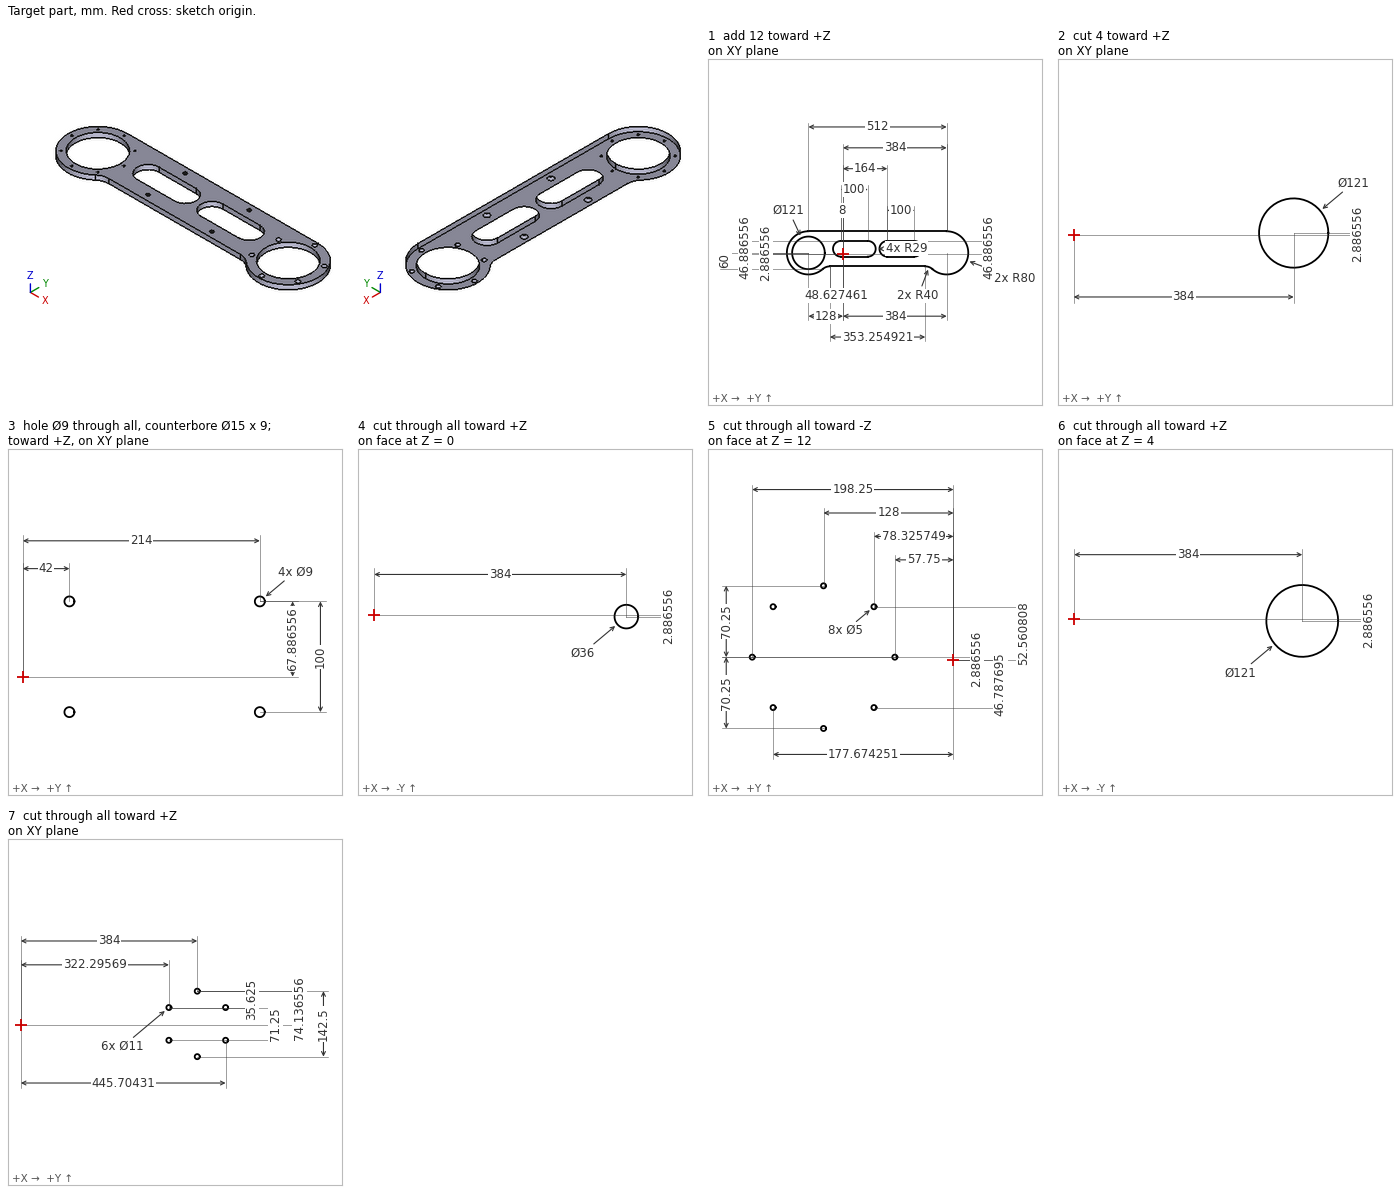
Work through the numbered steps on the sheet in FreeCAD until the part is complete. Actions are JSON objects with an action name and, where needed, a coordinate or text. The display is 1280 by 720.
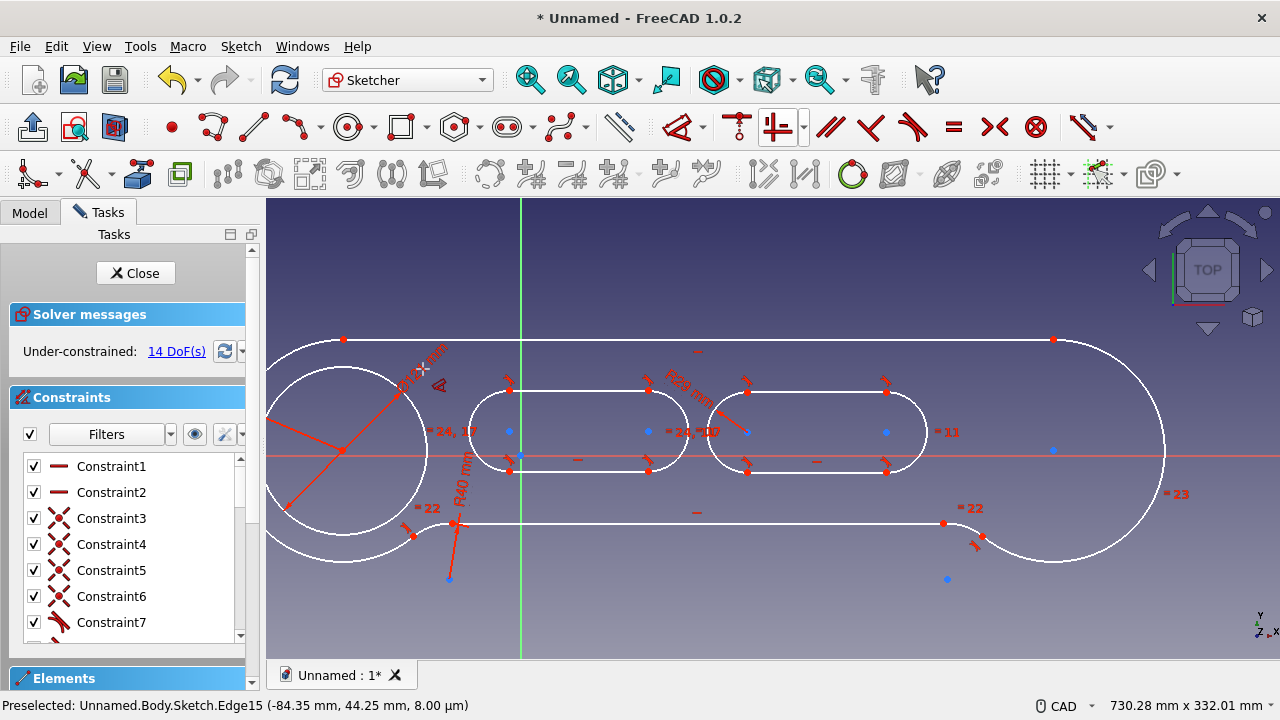
{"action": "scroll", "coordinate": [509, 391], "scroll_direction": "up", "scroll_amount": 7}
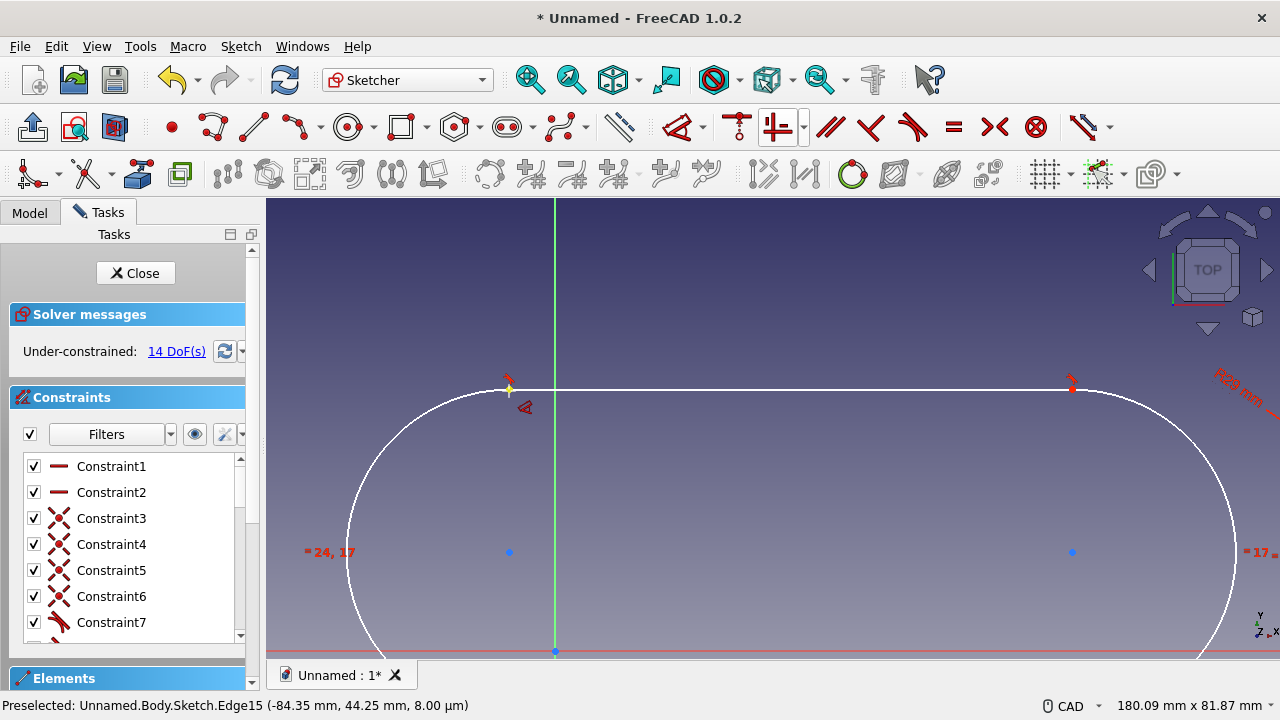
{"action": "left_click", "coordinate": [510, 390]}
{"action": "left_click", "coordinate": [533, 356]}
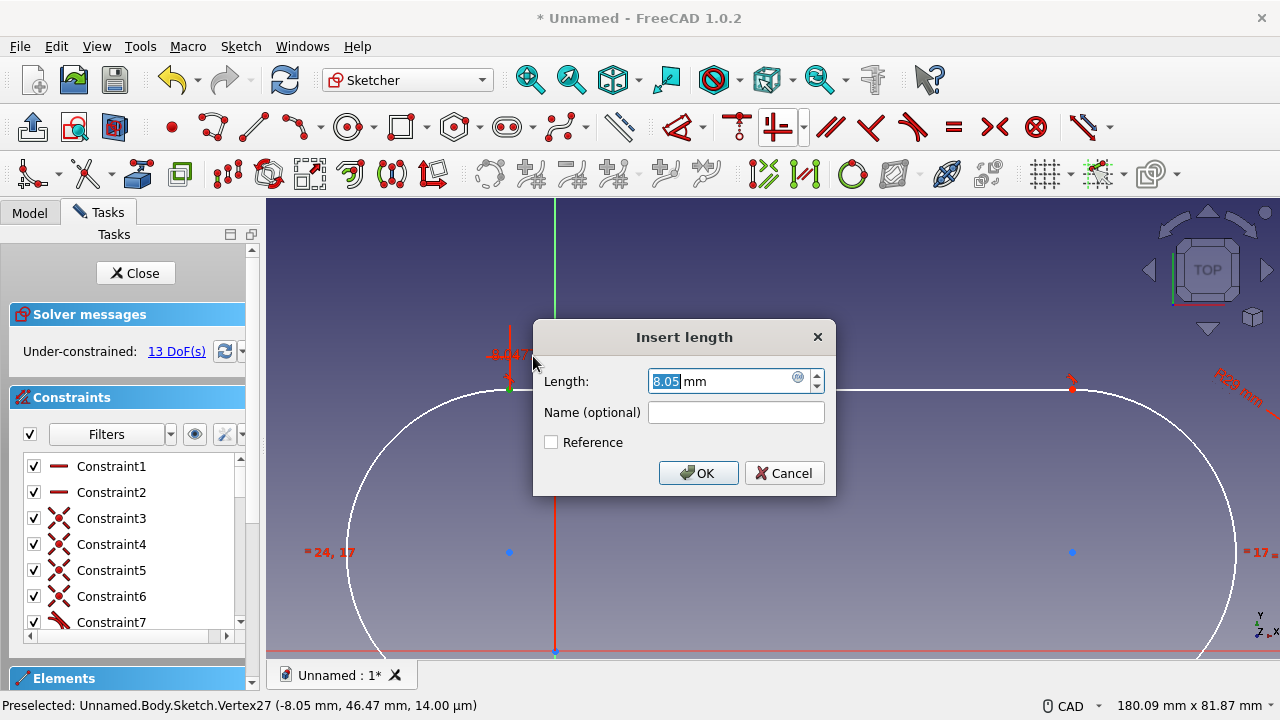
{"action": "type", "text": "8"}
{"action": "key", "text": "Return"}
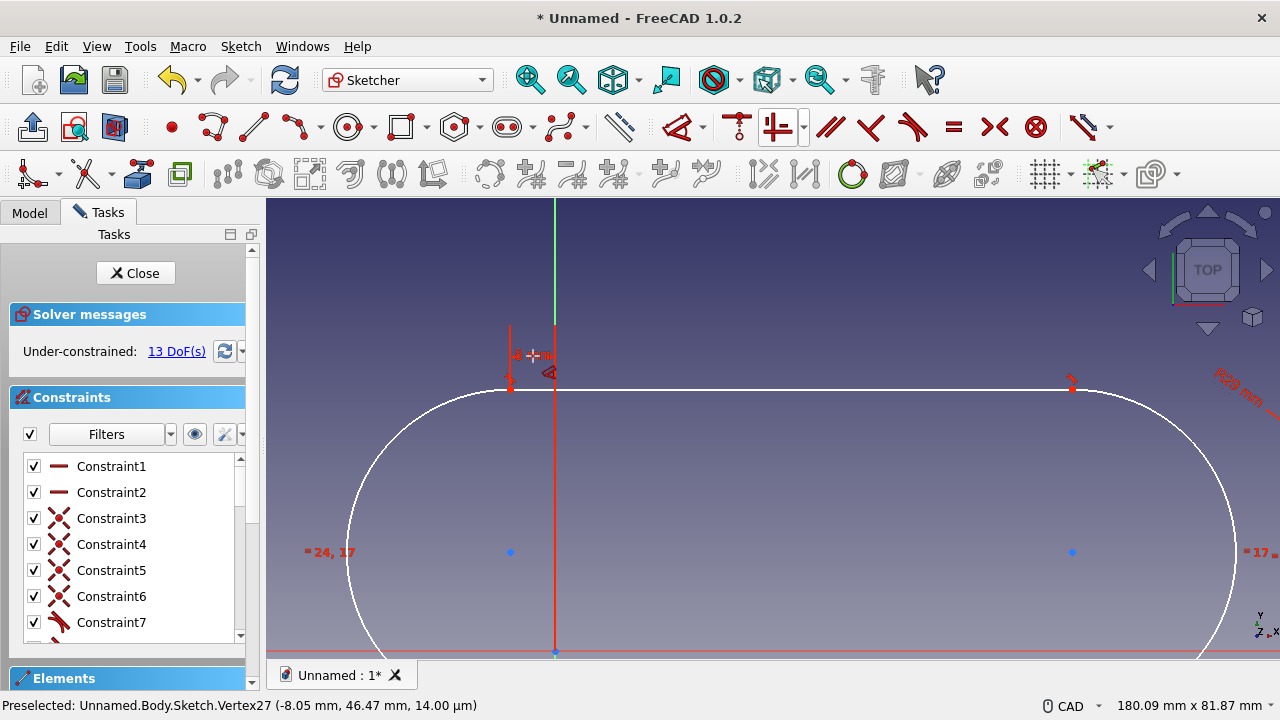
{"action": "scroll", "coordinate": [591, 398], "scroll_direction": "down", "scroll_amount": 9}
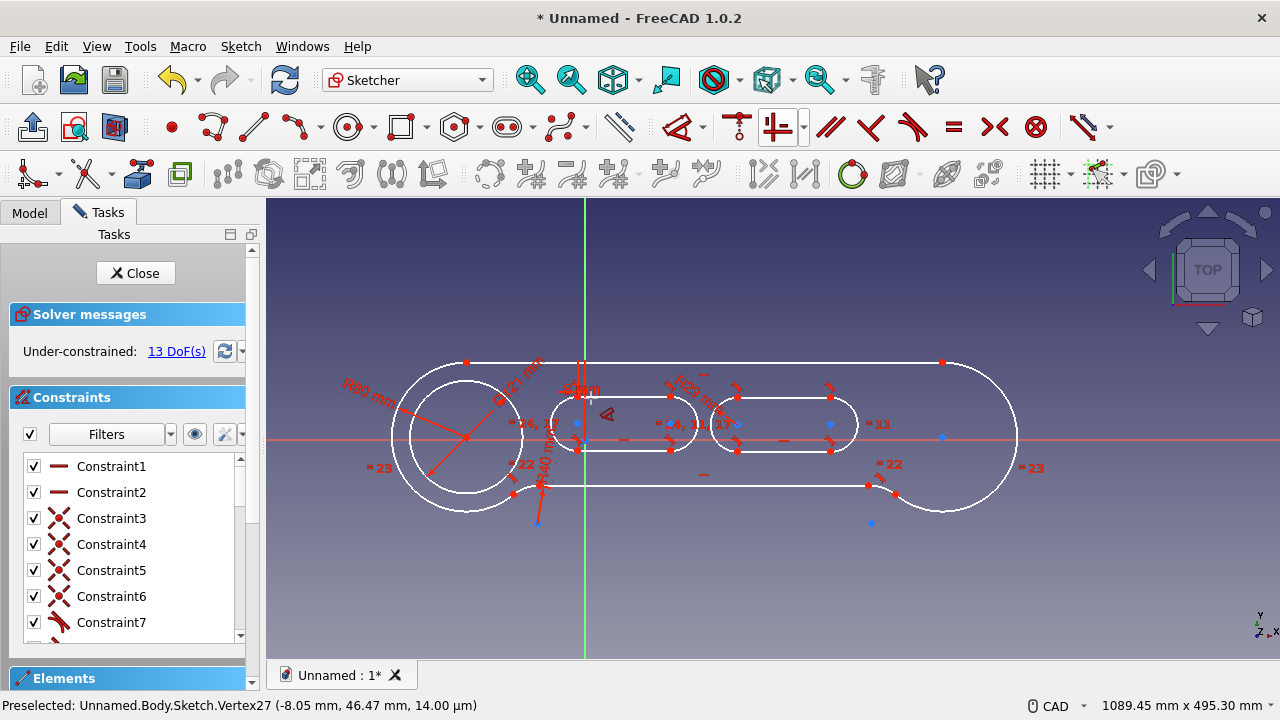
{"action": "left_click", "coordinate": [800, 363]}
{"action": "left_click", "coordinate": [705, 329]}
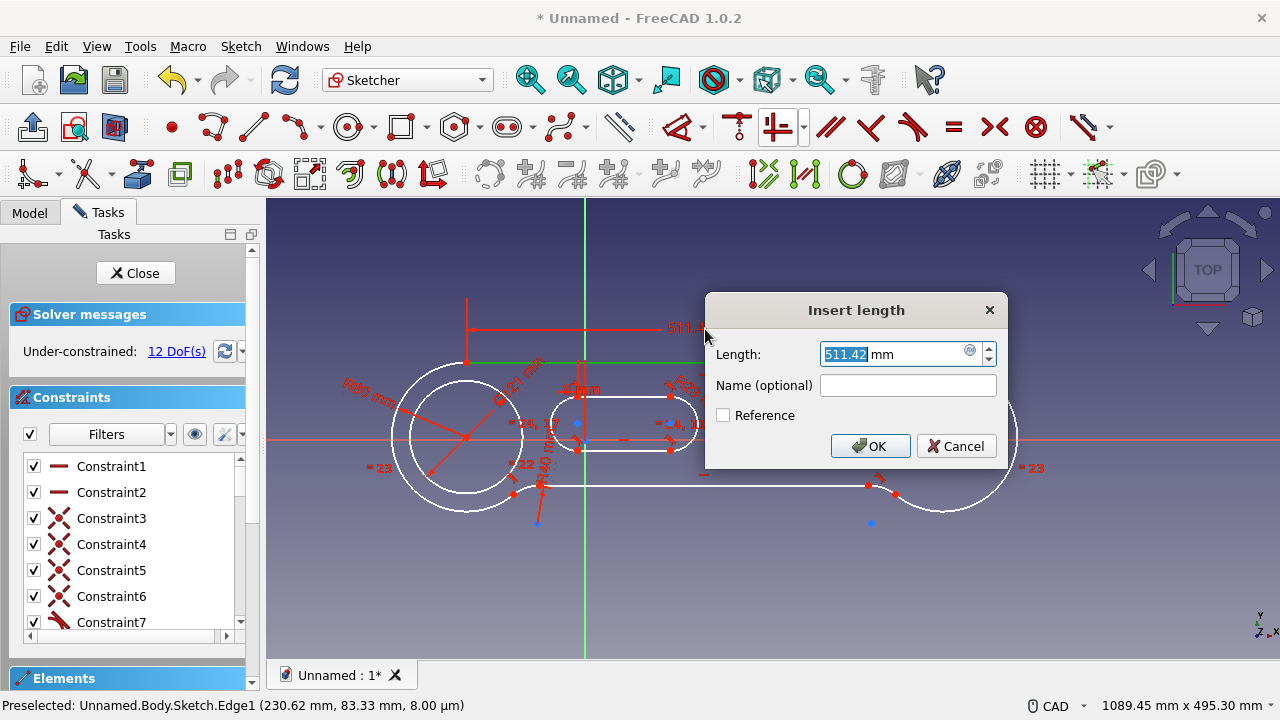
{"action": "type", "text": "512"}
{"action": "key", "text": "Return"}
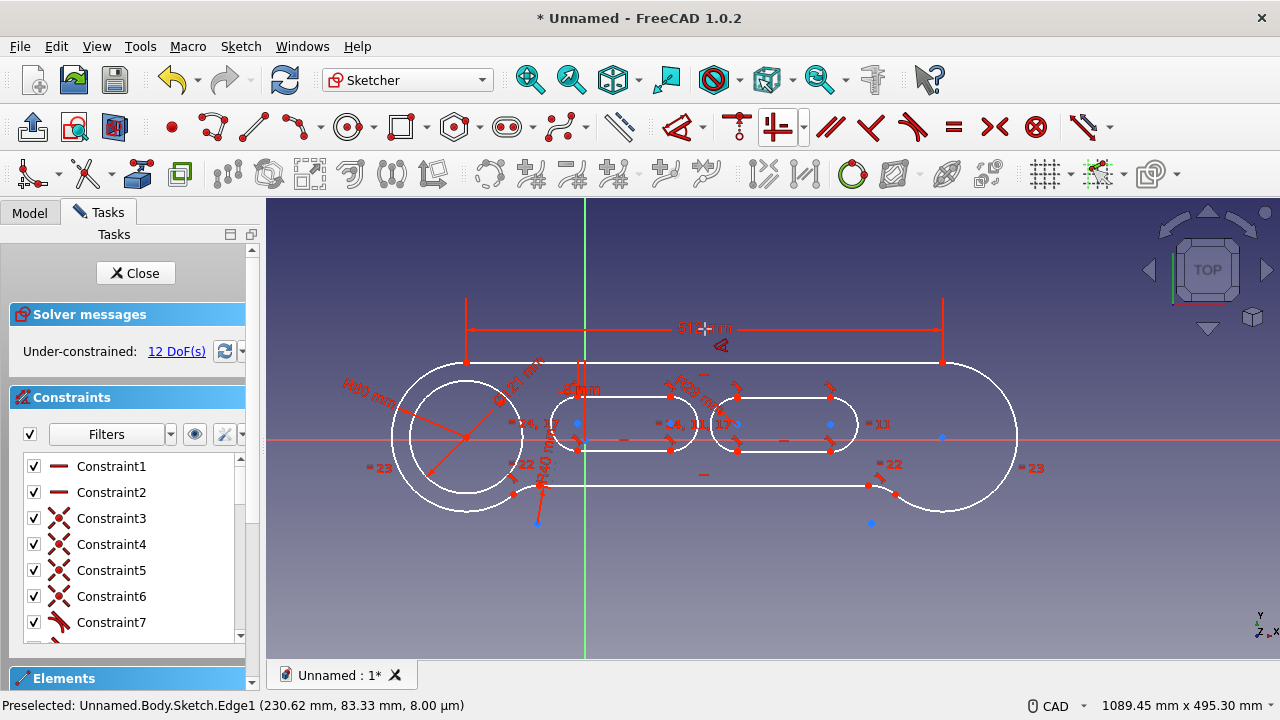
{"action": "left_click", "coordinate": [766, 398]}
{"action": "left_click", "coordinate": [784, 340]}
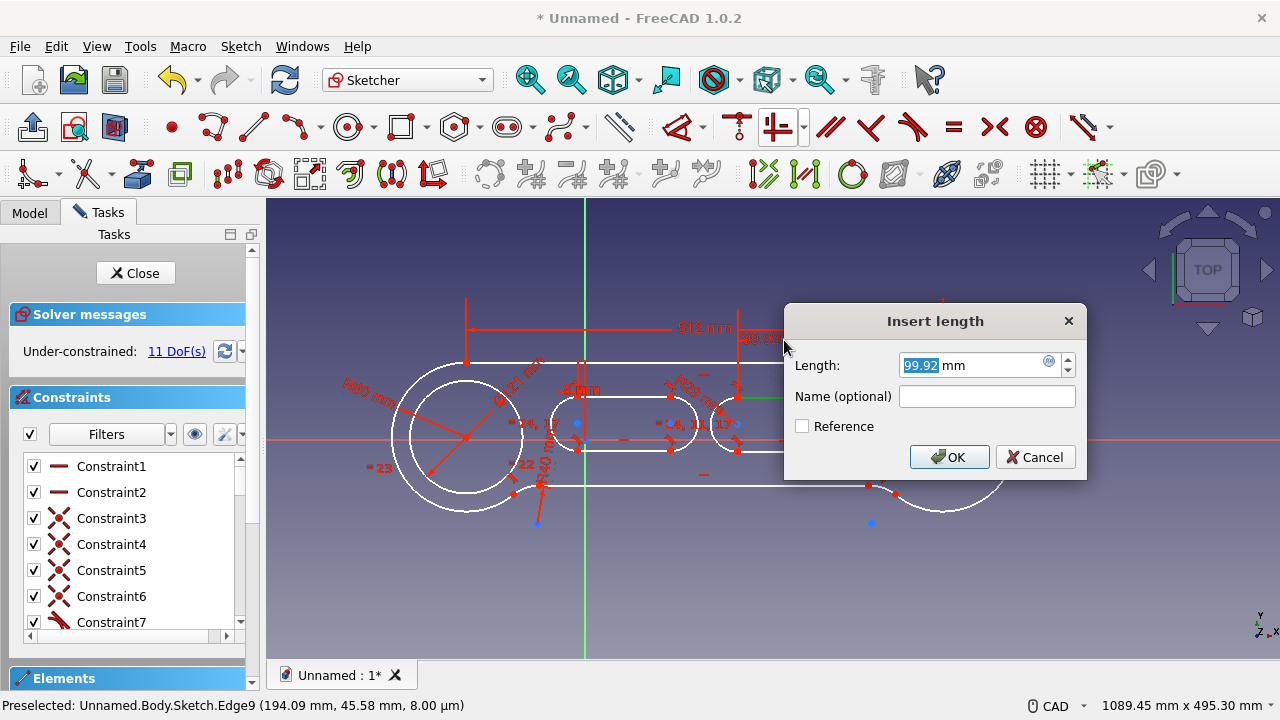
{"action": "type", "text": "100"}
{"action": "key", "text": "Return"}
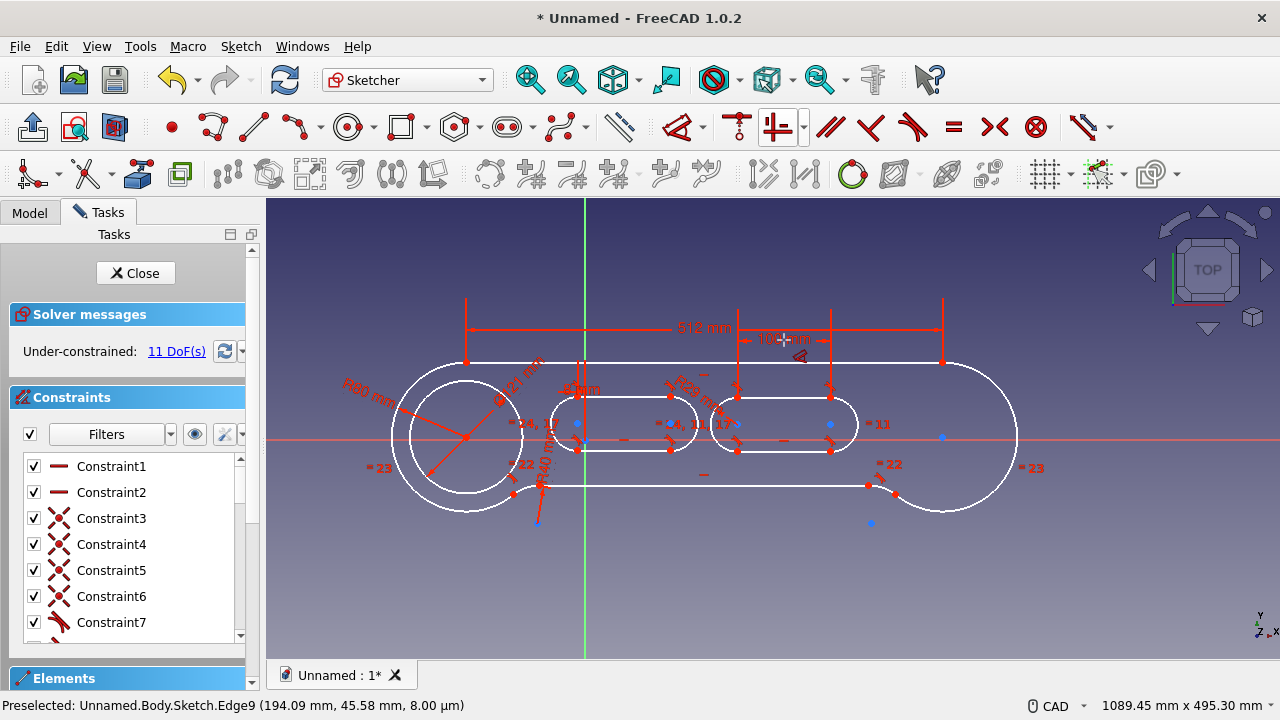
{"action": "left_click", "coordinate": [606, 397]}
{"action": "left_click", "coordinate": [624, 339]}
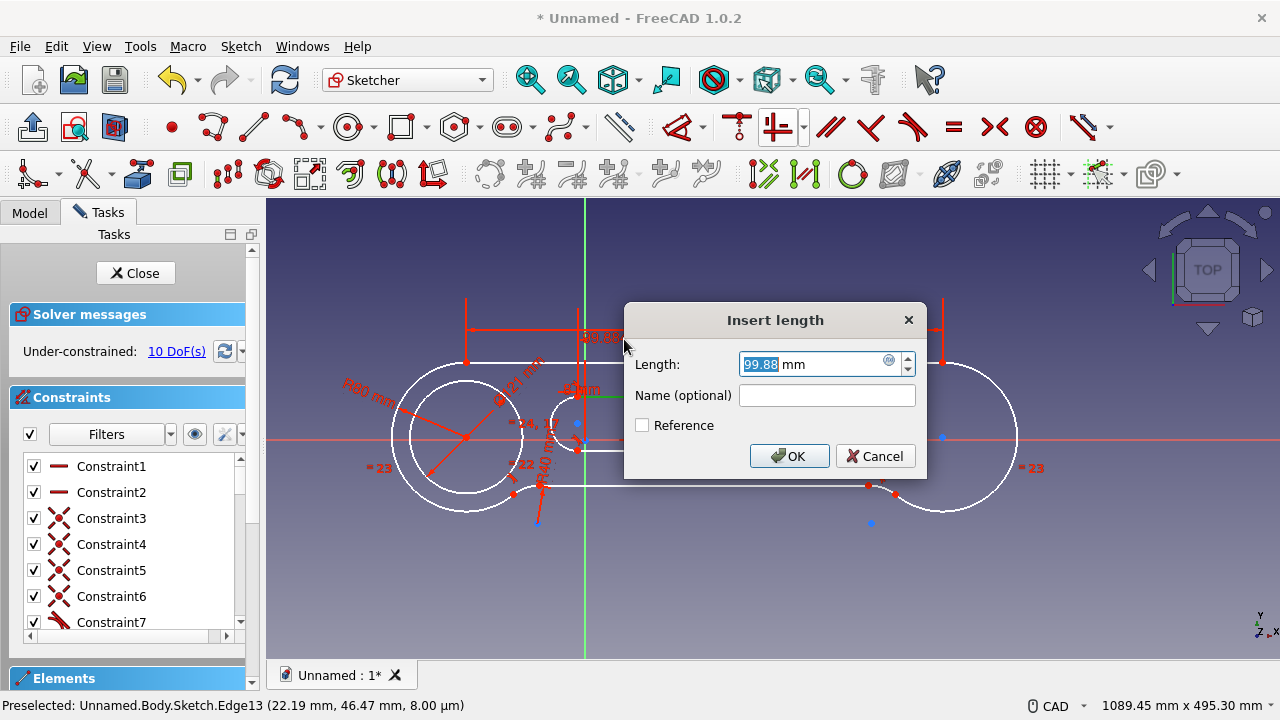
{"action": "type", "text": "100"}
{"action": "key", "text": "Return"}